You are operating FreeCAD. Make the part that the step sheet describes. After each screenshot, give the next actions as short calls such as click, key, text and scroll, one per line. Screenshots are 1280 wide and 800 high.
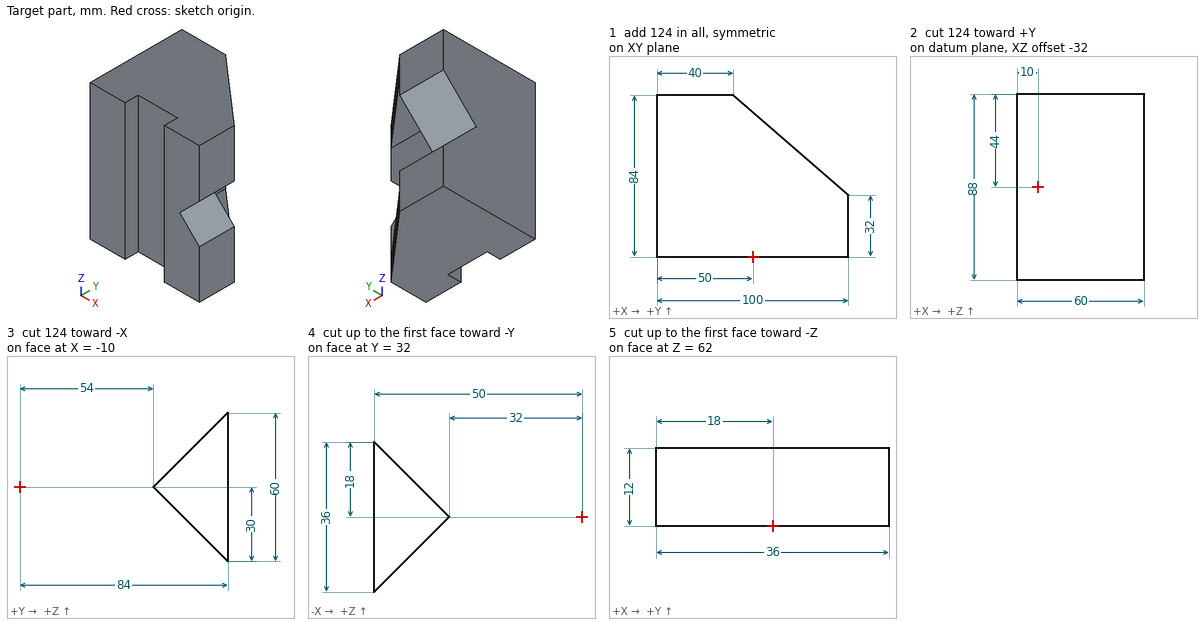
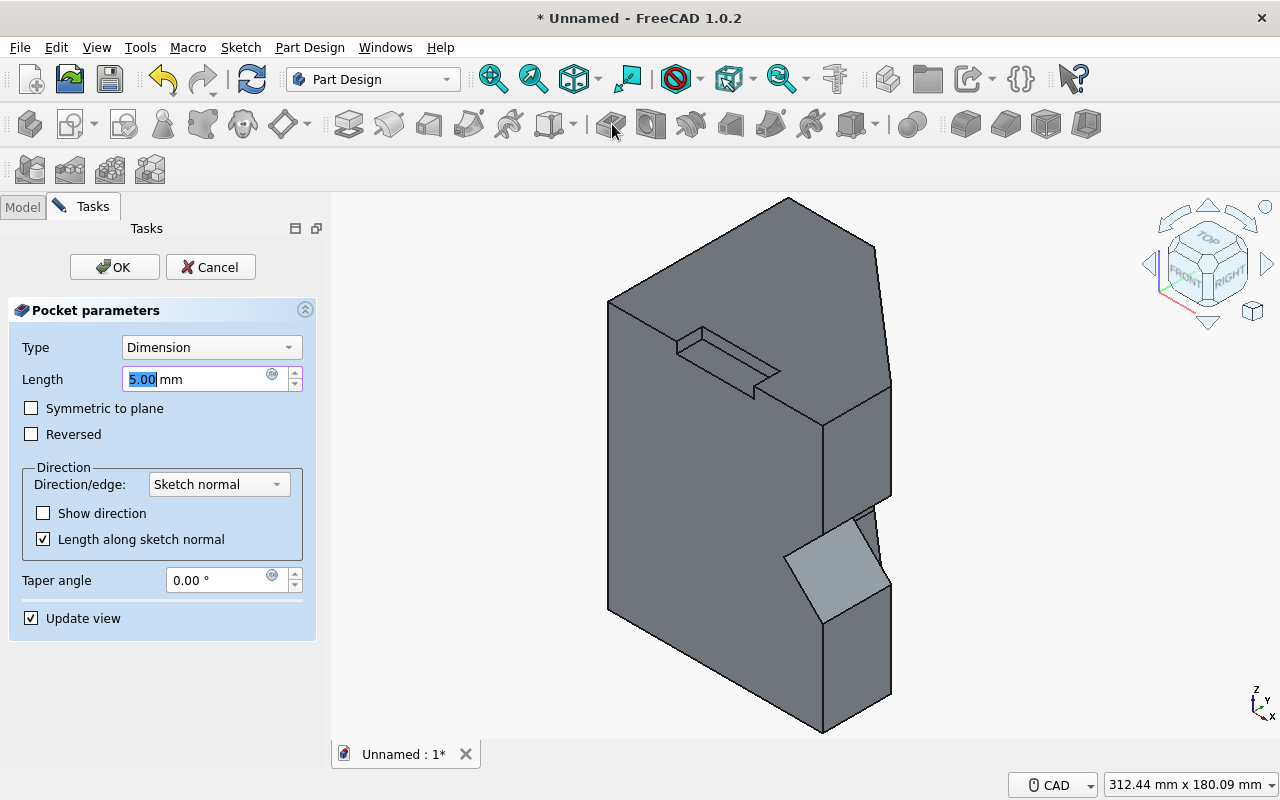
click(212, 348)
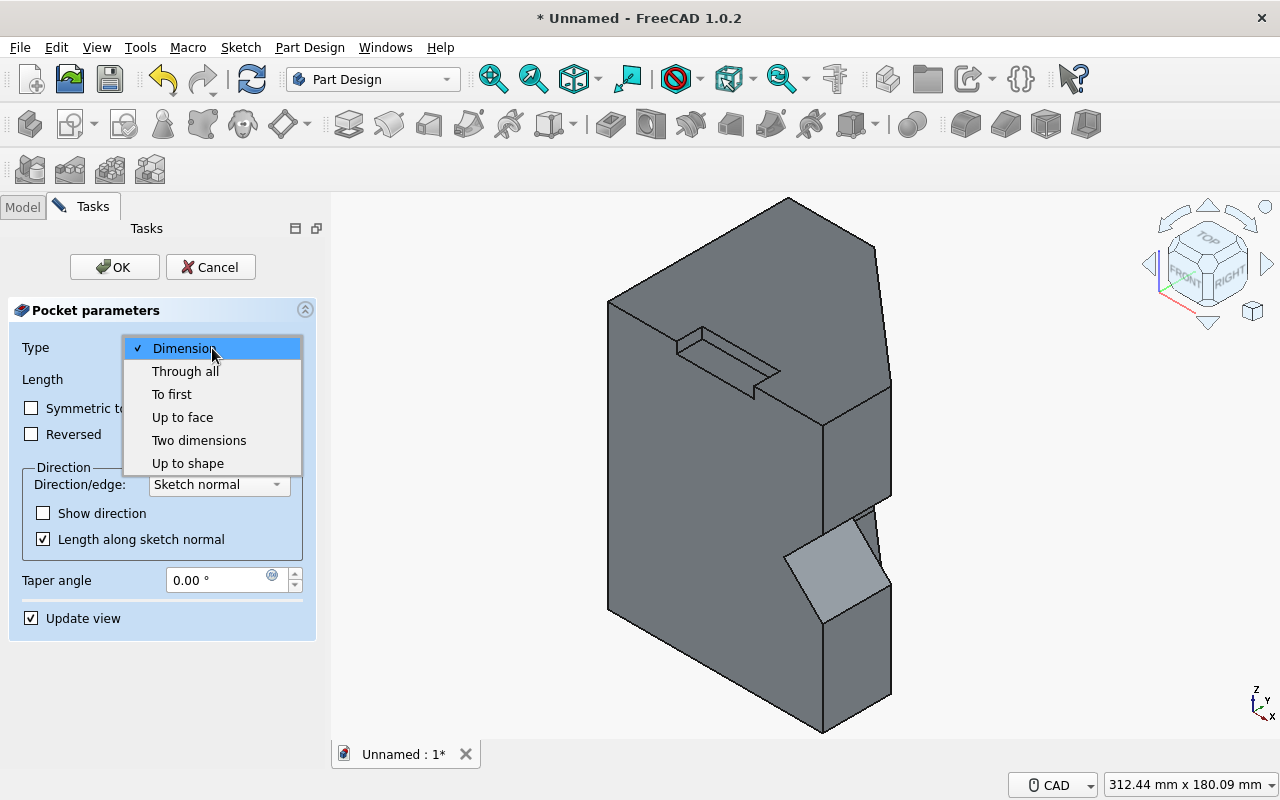
click(212, 394)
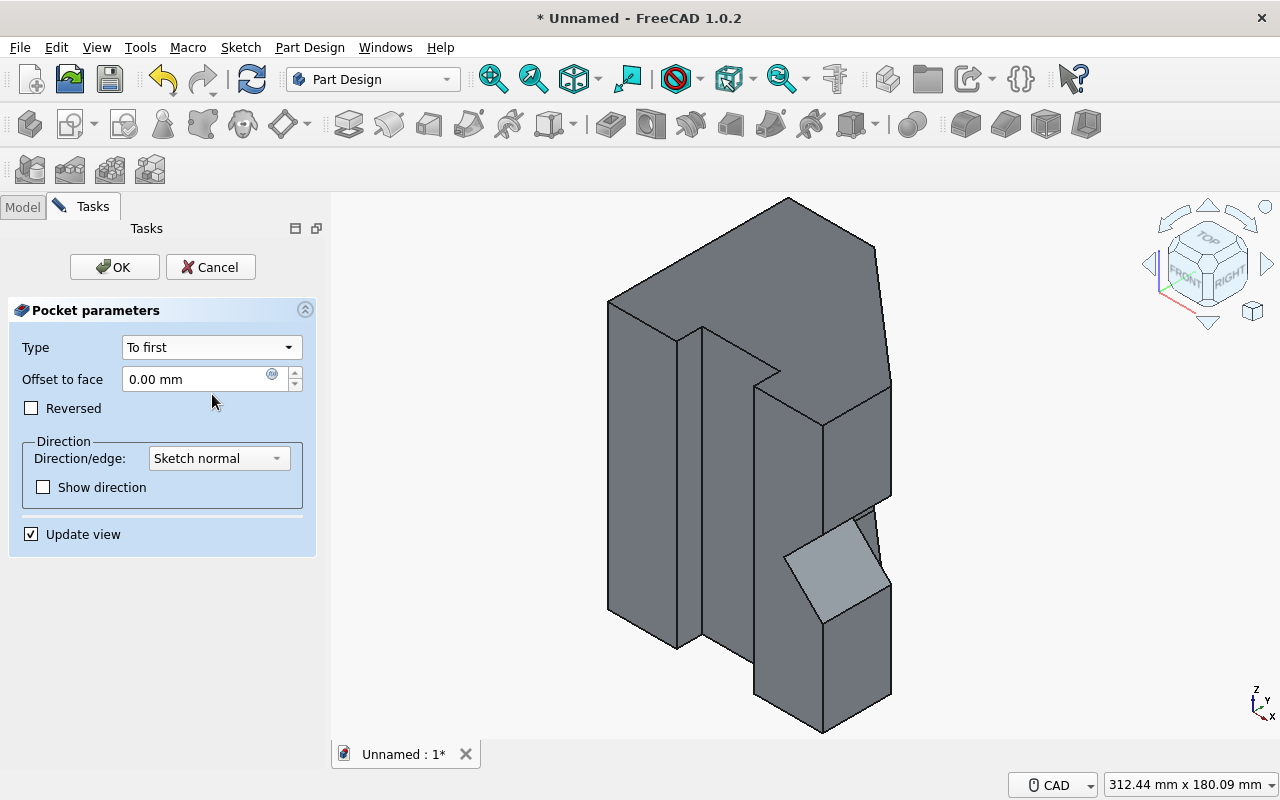
click(115, 267)